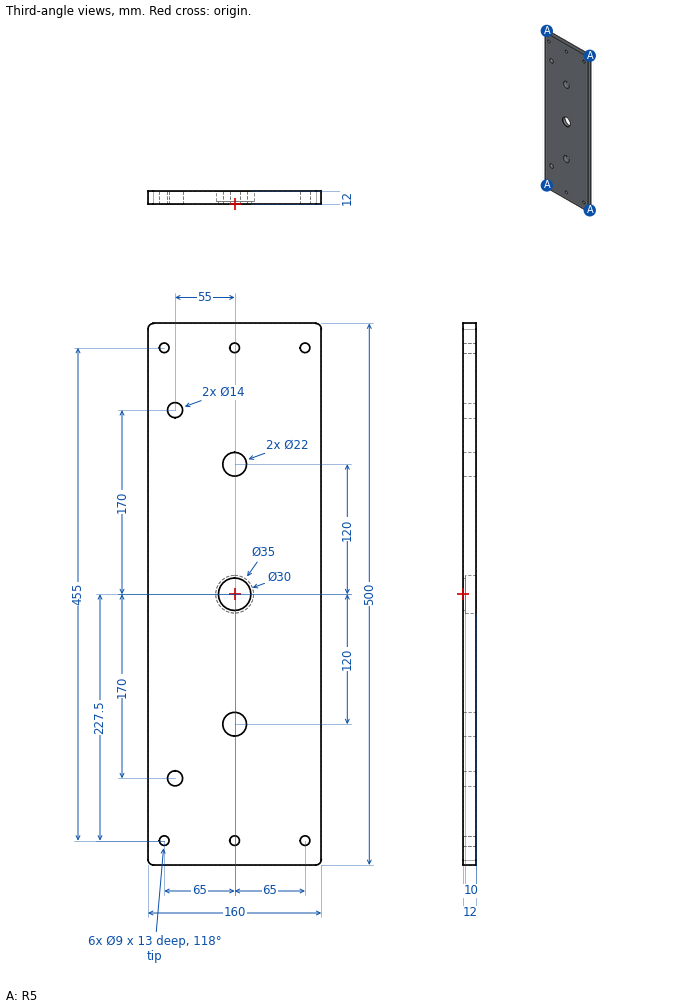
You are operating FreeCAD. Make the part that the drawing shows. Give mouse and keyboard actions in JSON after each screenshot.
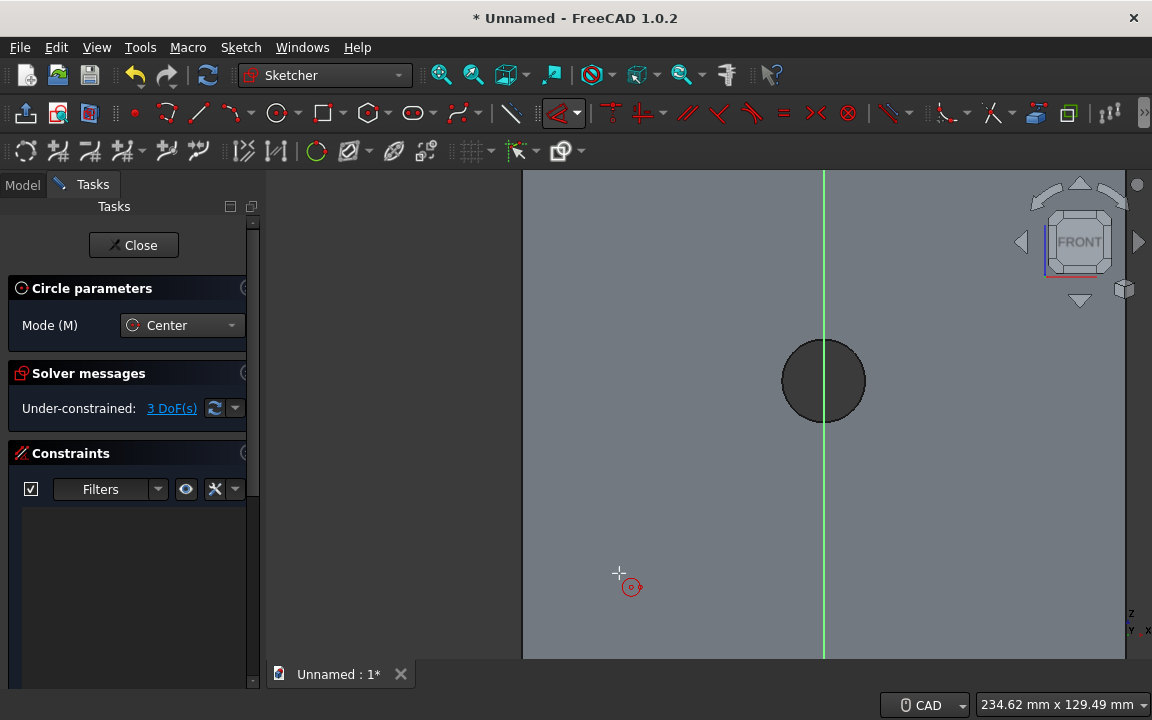
{"action": "scroll", "coordinate": [619, 574], "scroll_direction": "down", "scroll_amount": 7}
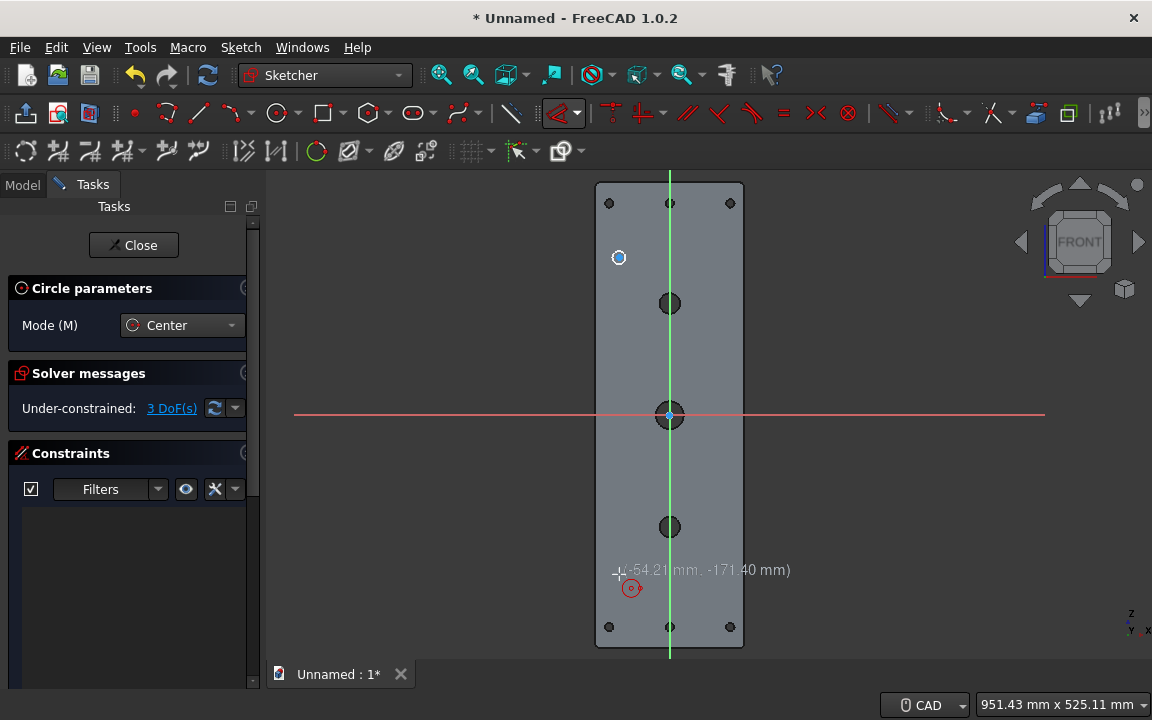
{"action": "left_click", "coordinate": [619, 574]}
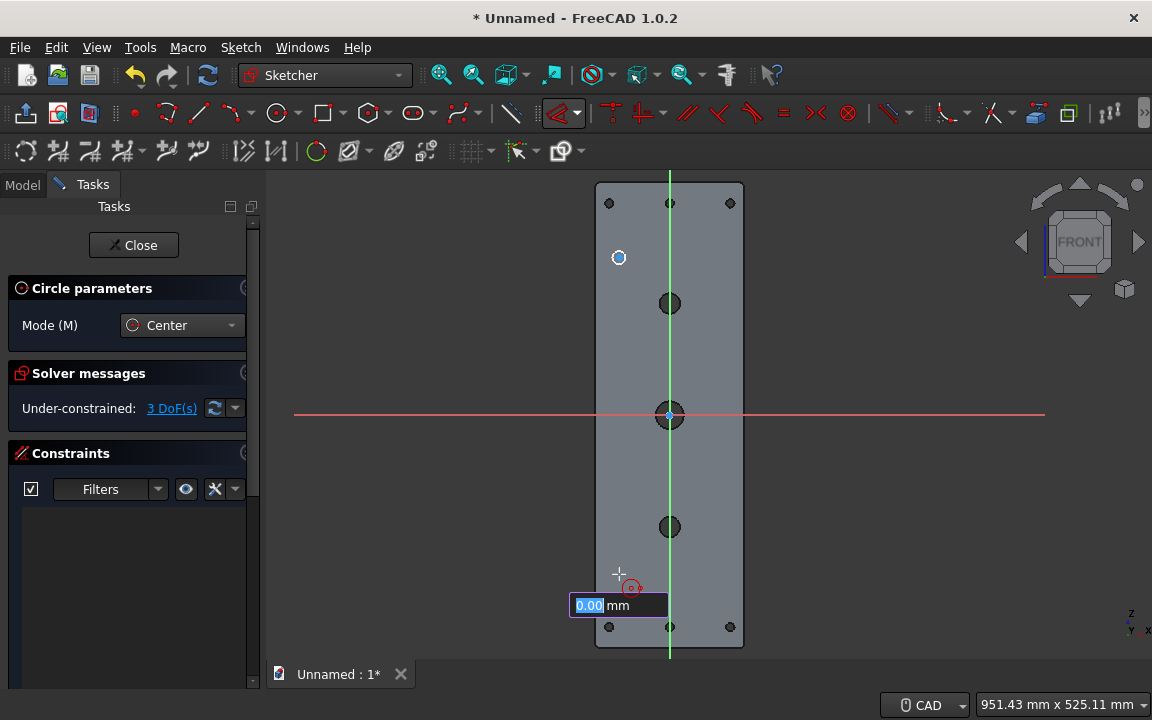
{"action": "scroll", "coordinate": [623, 569], "scroll_direction": "up", "scroll_amount": 5}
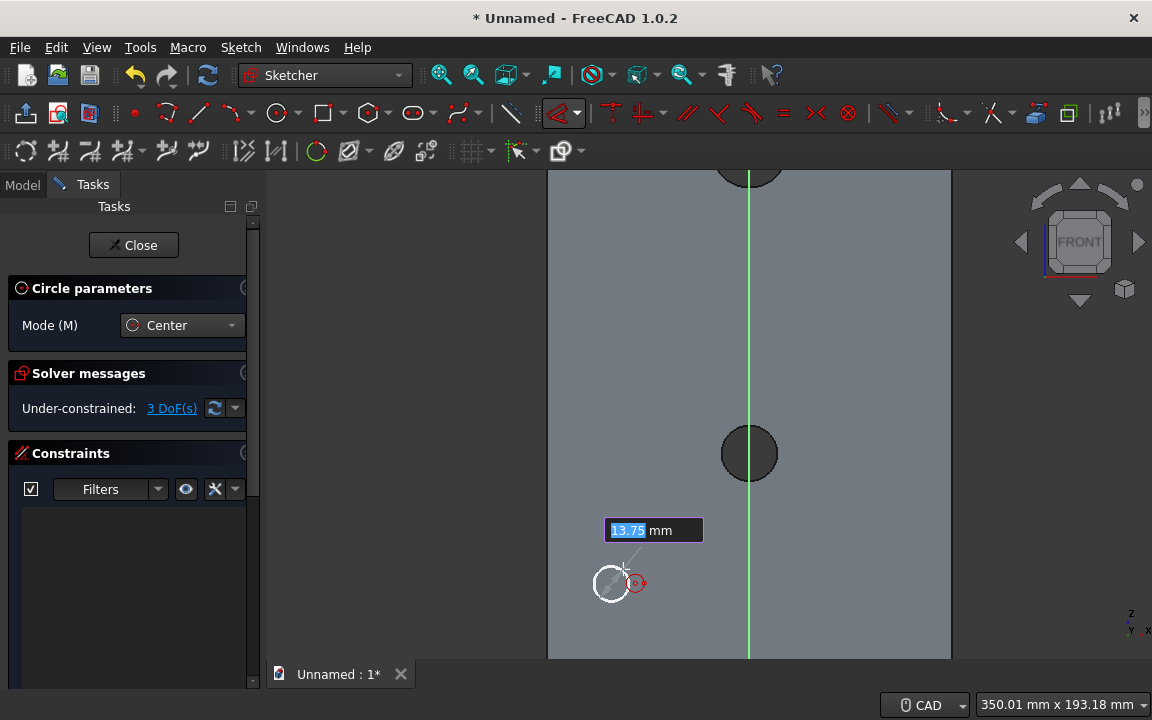
{"action": "left_click", "coordinate": [623, 567]}
{"action": "key", "text": "Escape"}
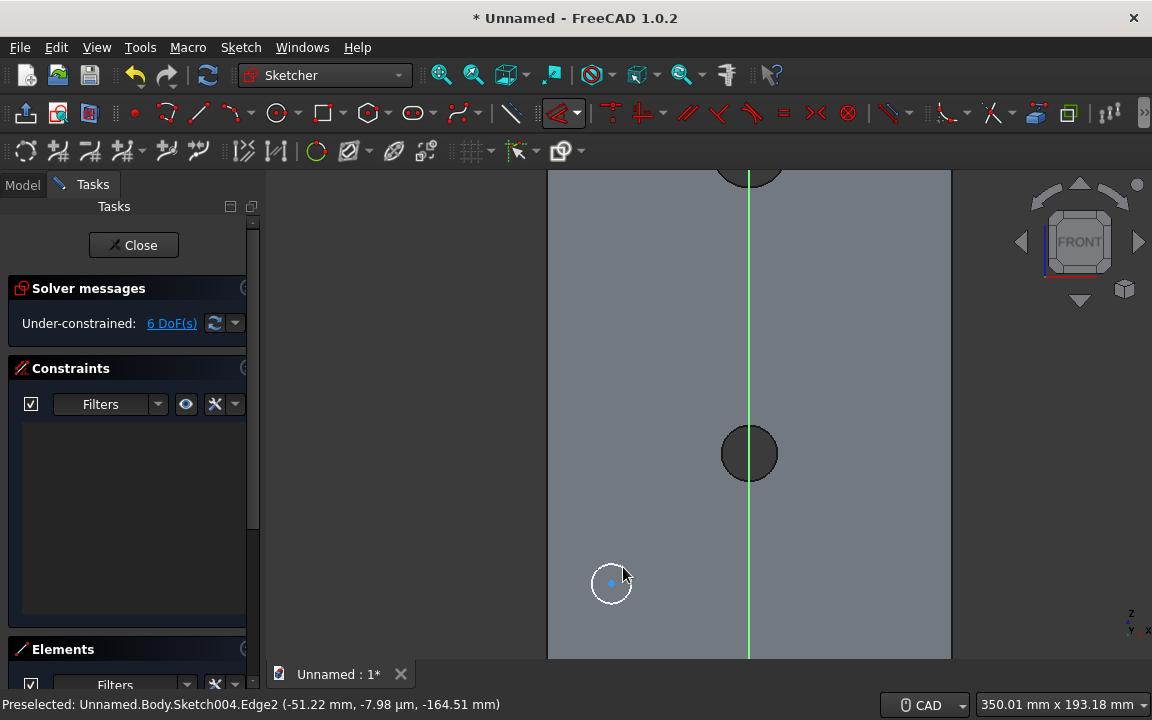
{"action": "scroll", "coordinate": [623, 569], "scroll_direction": "down", "scroll_amount": 5}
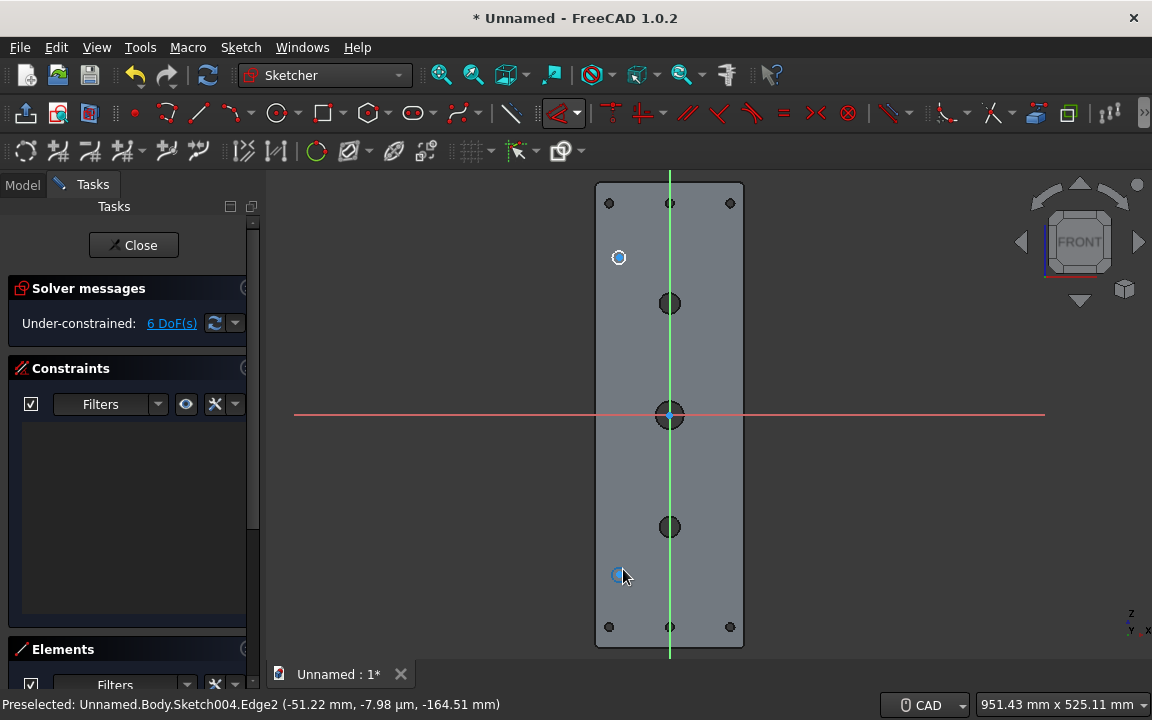
{"action": "scroll", "coordinate": [624, 253], "scroll_direction": "up", "scroll_amount": 4}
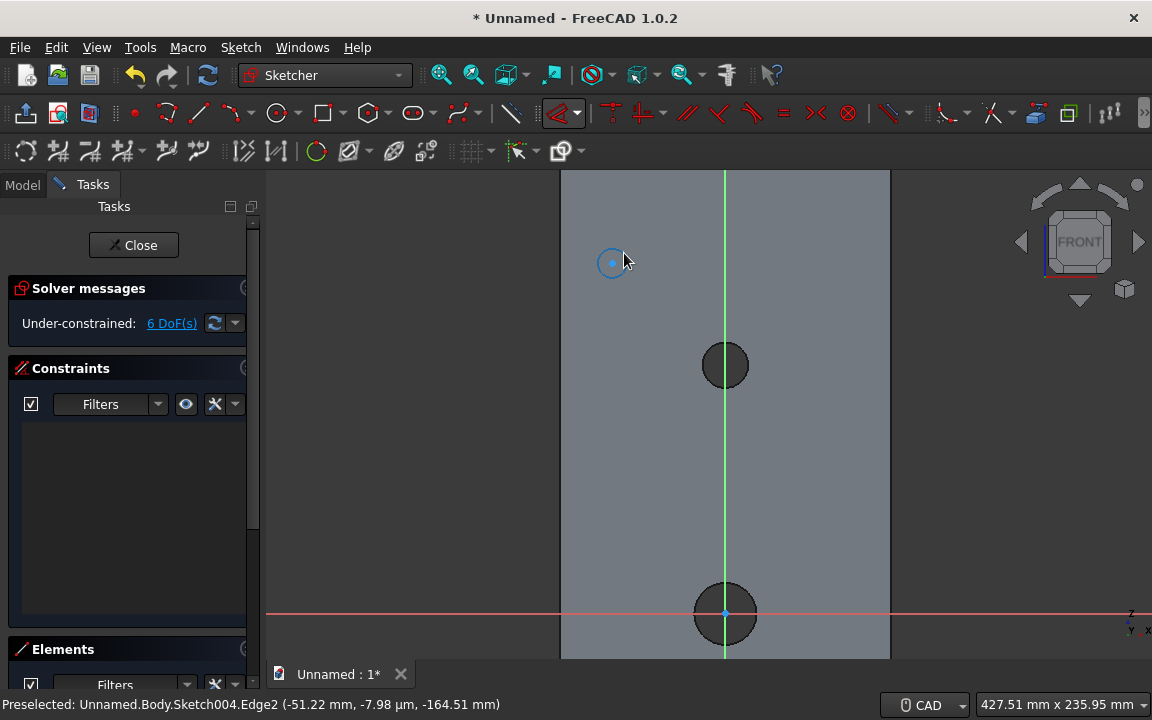
{"action": "left_click", "coordinate": [623, 253]}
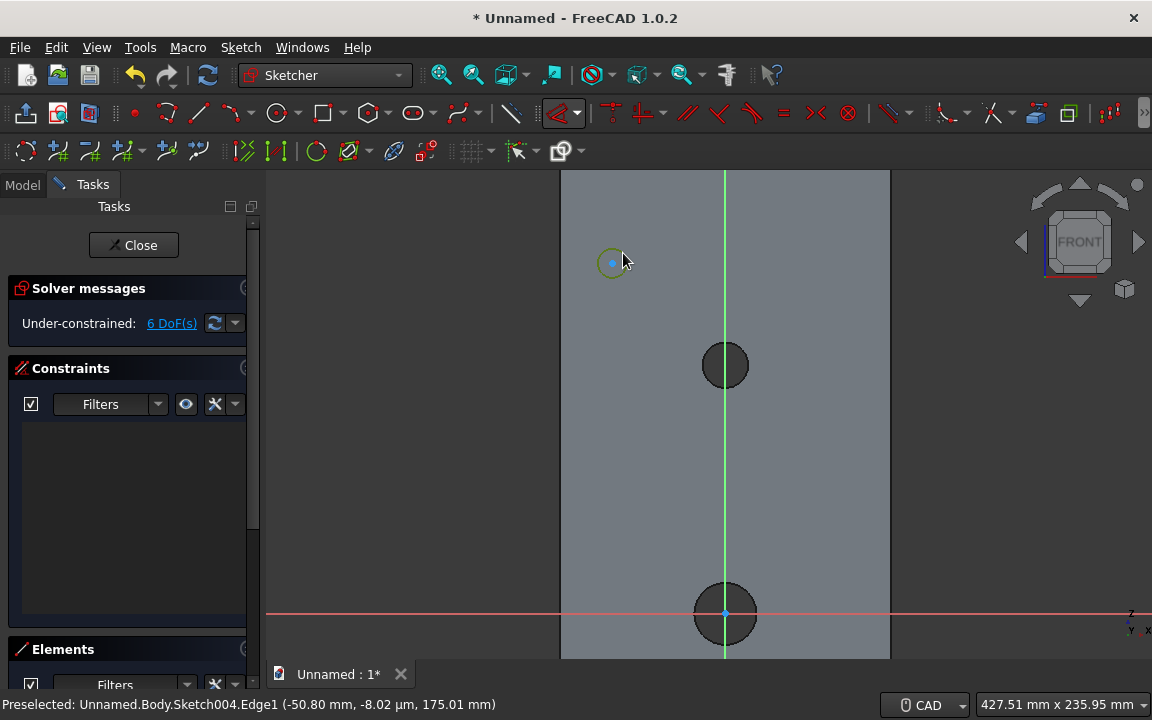
{"action": "scroll", "coordinate": [624, 252], "scroll_direction": "down", "scroll_amount": 4}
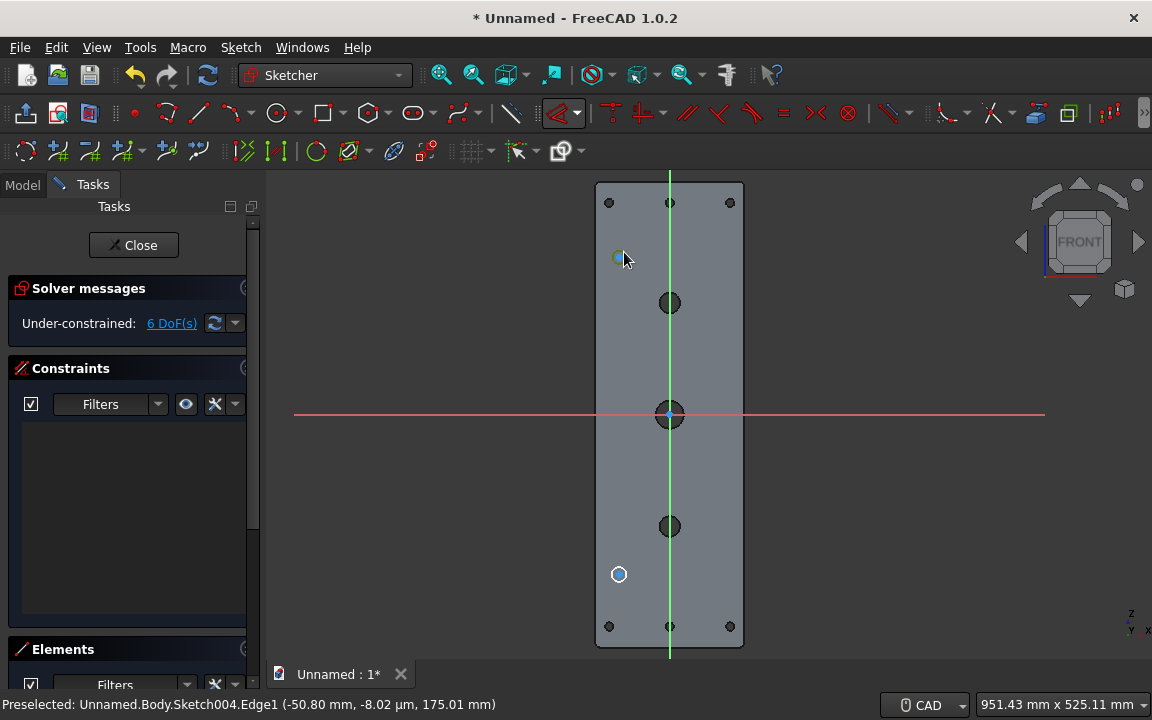
{"action": "scroll", "coordinate": [624, 569], "scroll_direction": "up", "scroll_amount": 4}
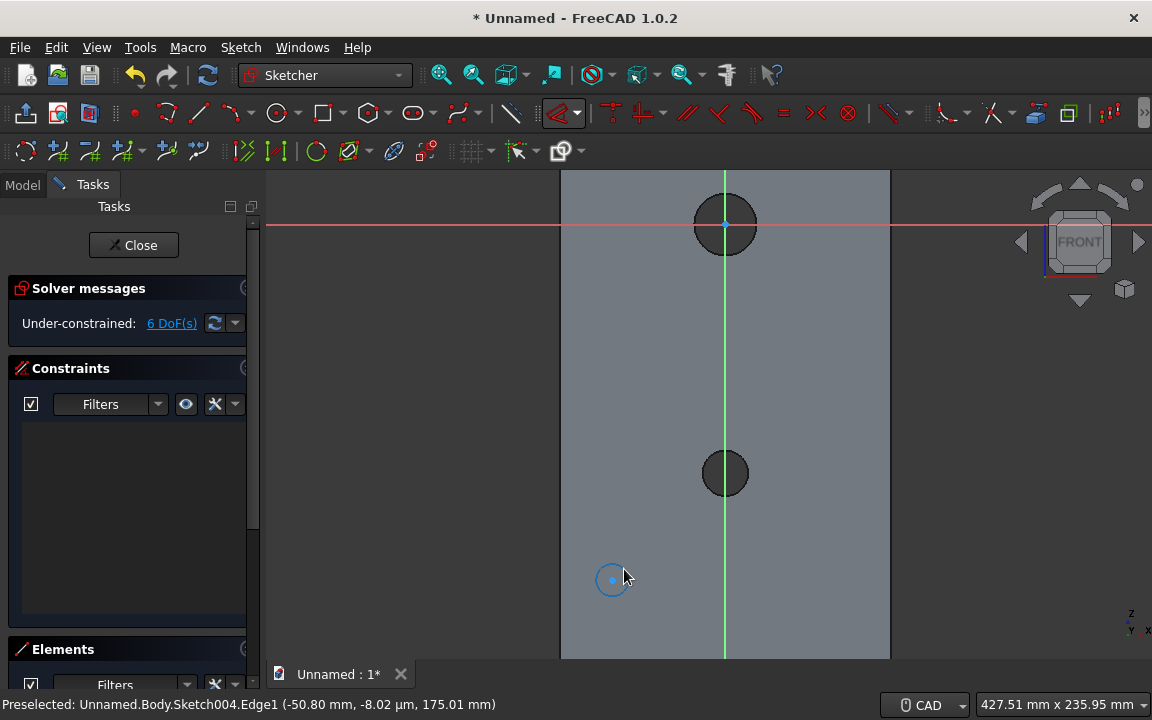
{"action": "left_click", "coordinate": [624, 569]}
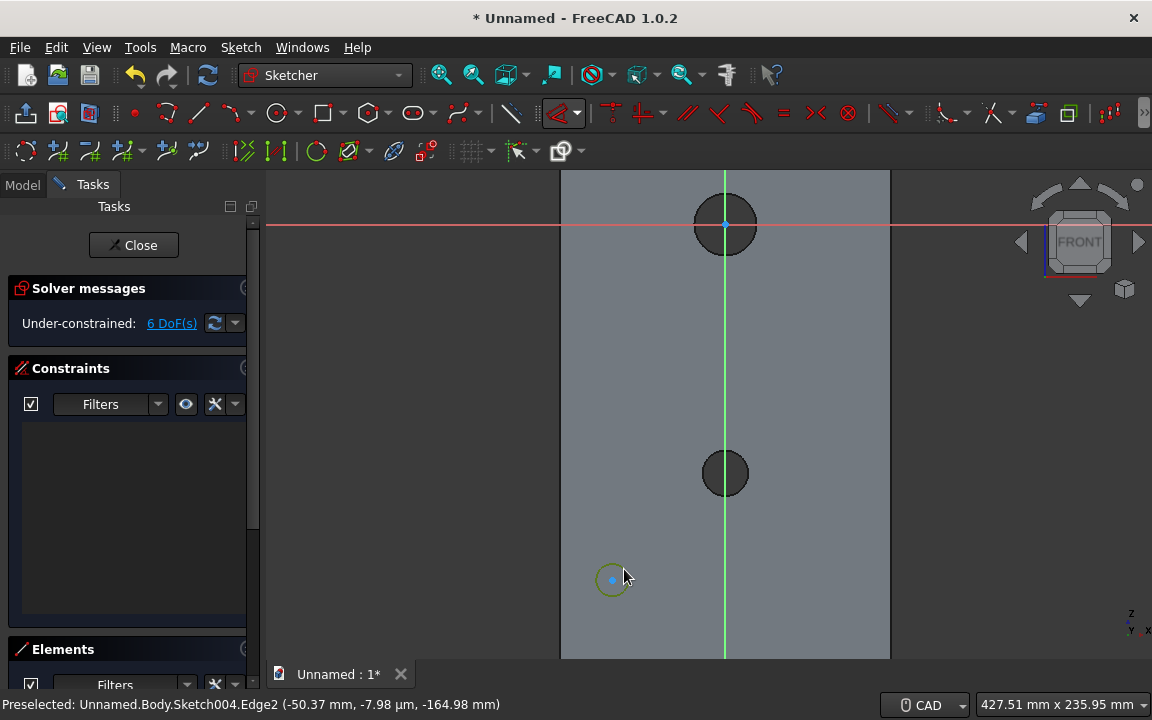
{"action": "left_click", "coordinate": [784, 114]}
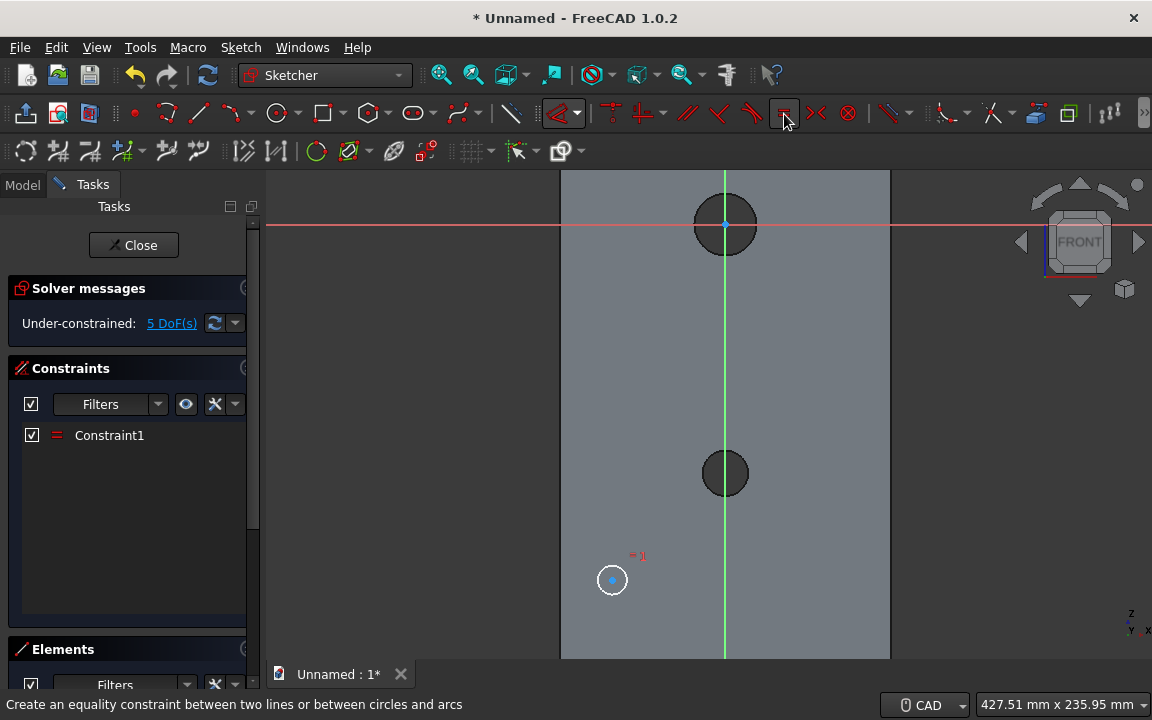
{"action": "scroll", "coordinate": [624, 569], "scroll_direction": "down", "scroll_amount": 4}